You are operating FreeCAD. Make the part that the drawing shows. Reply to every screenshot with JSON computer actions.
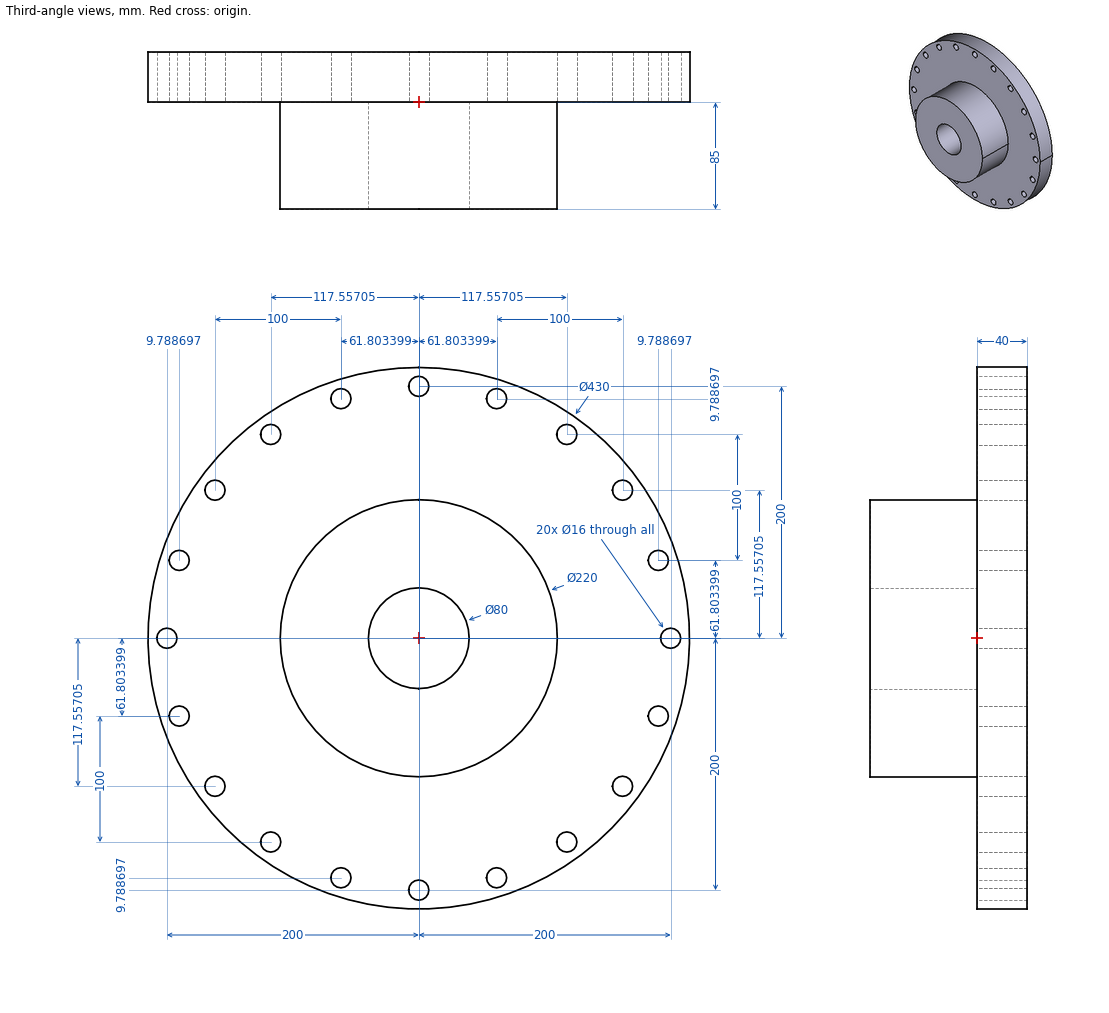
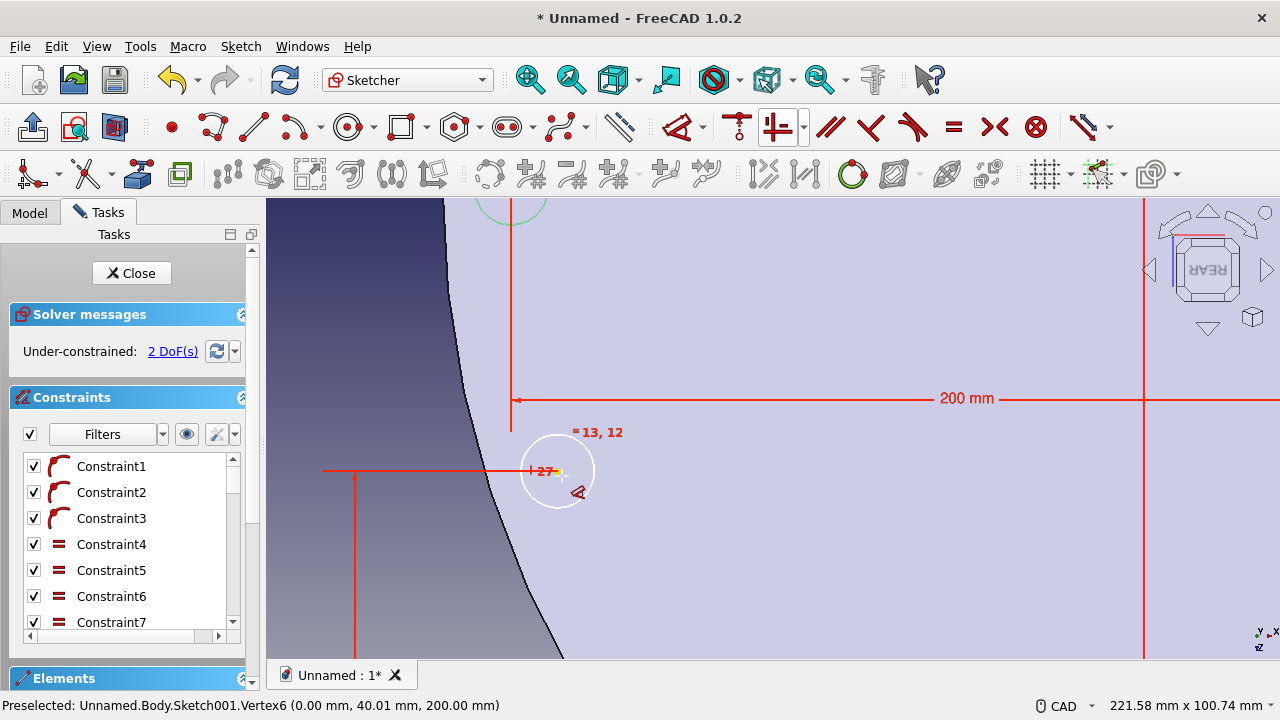
{"action": "left_click", "coordinate": [558, 471]}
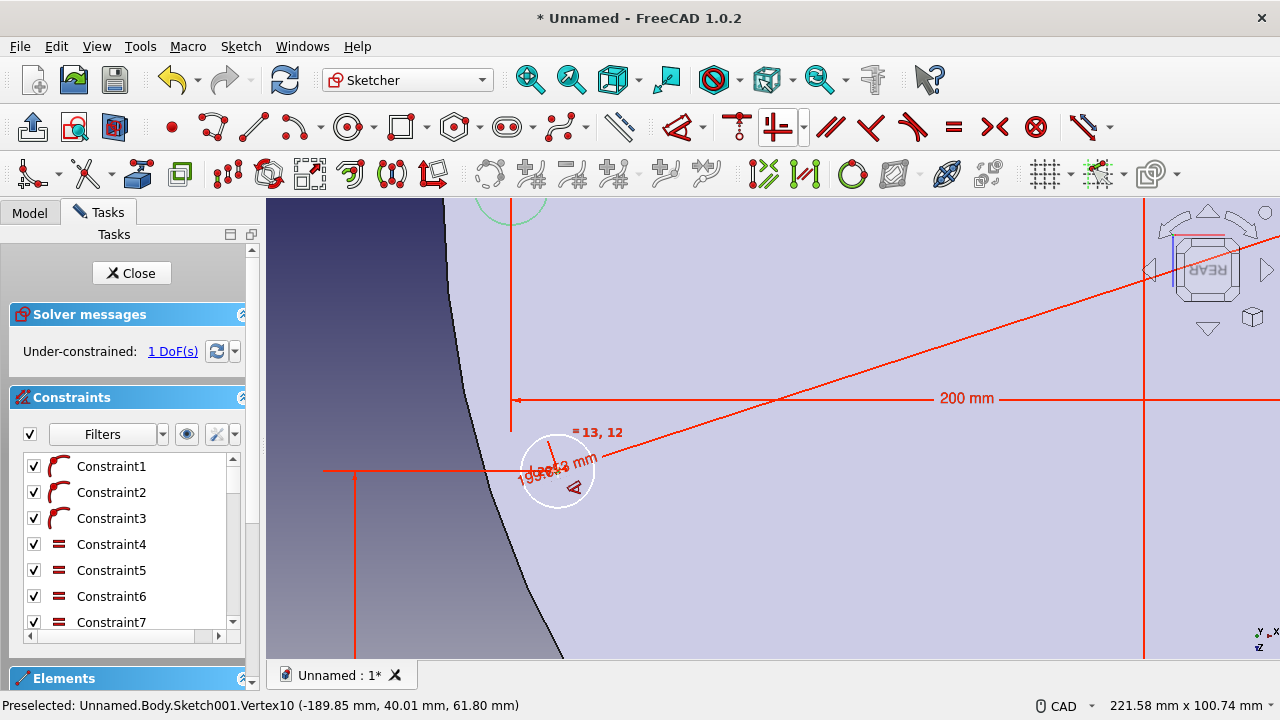
{"action": "scroll", "coordinate": [562, 476], "scroll_direction": "down", "scroll_amount": 9}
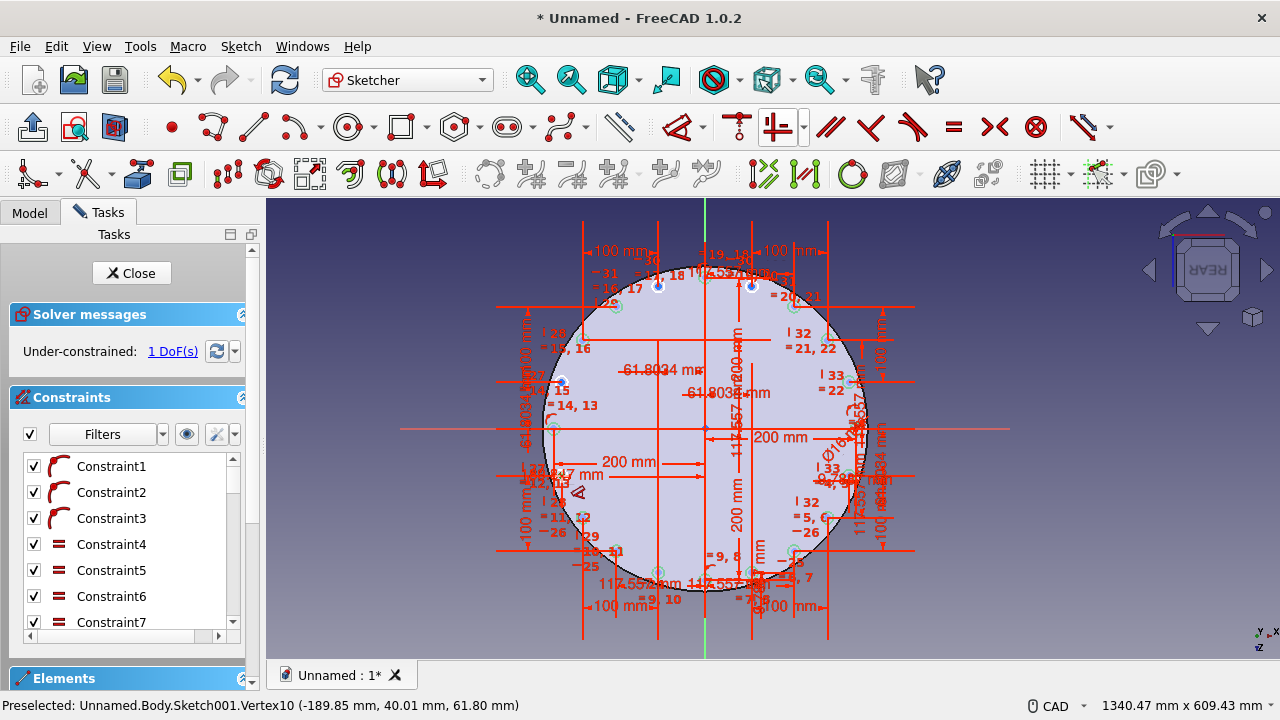
{"action": "scroll", "coordinate": [554, 429], "scroll_direction": "up", "scroll_amount": 9}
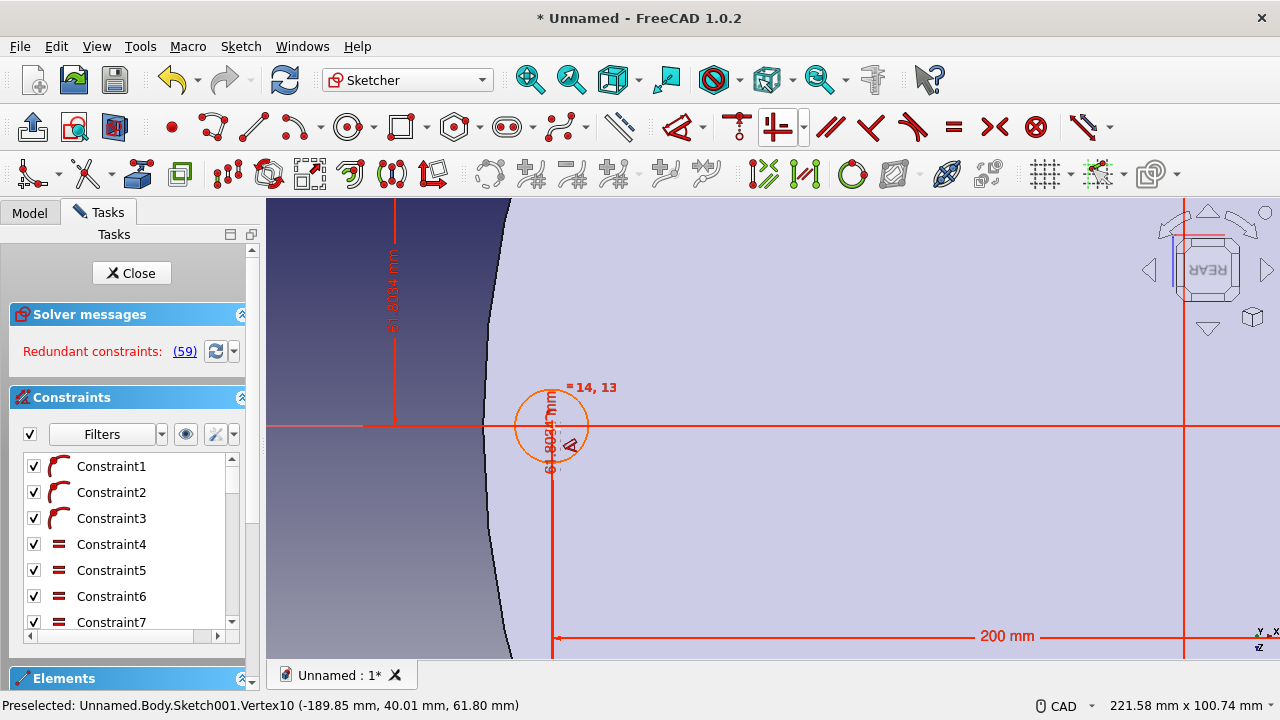
{"action": "left_click", "coordinate": [552, 426]}
{"action": "left_click", "coordinate": [591, 392]}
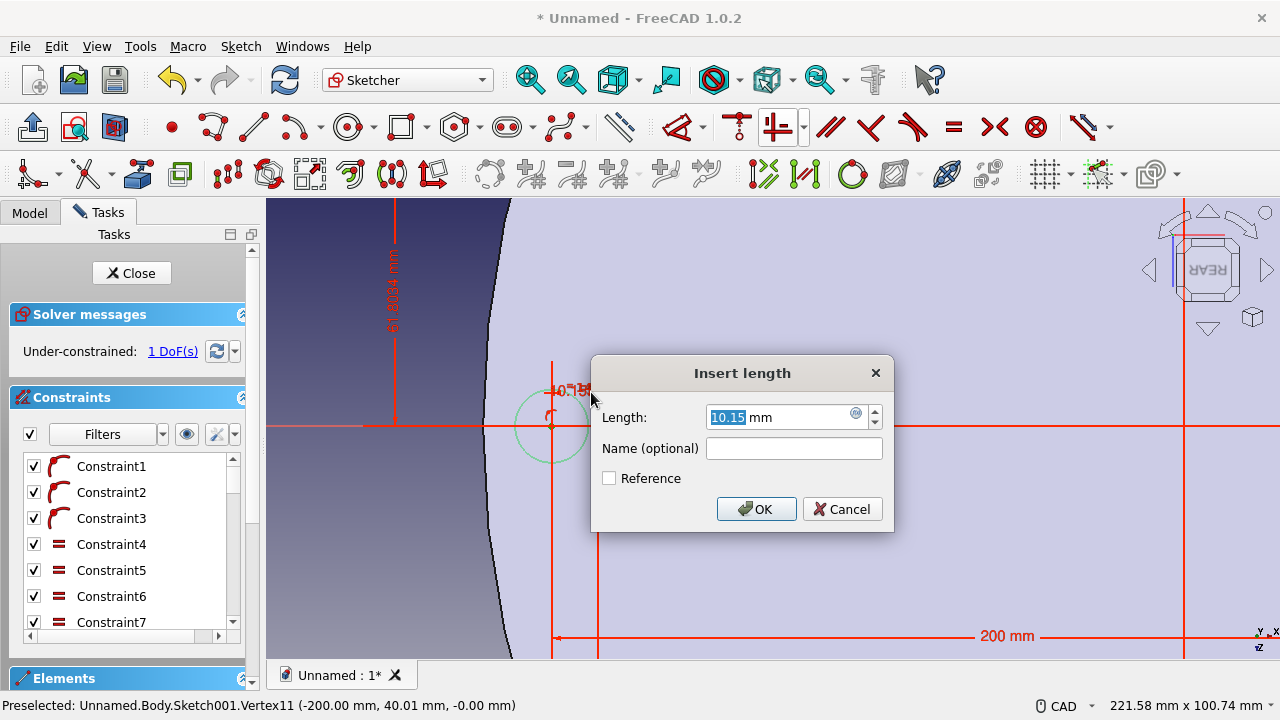
{"action": "type", "text": "9.788697"}
{"action": "key", "text": "Return"}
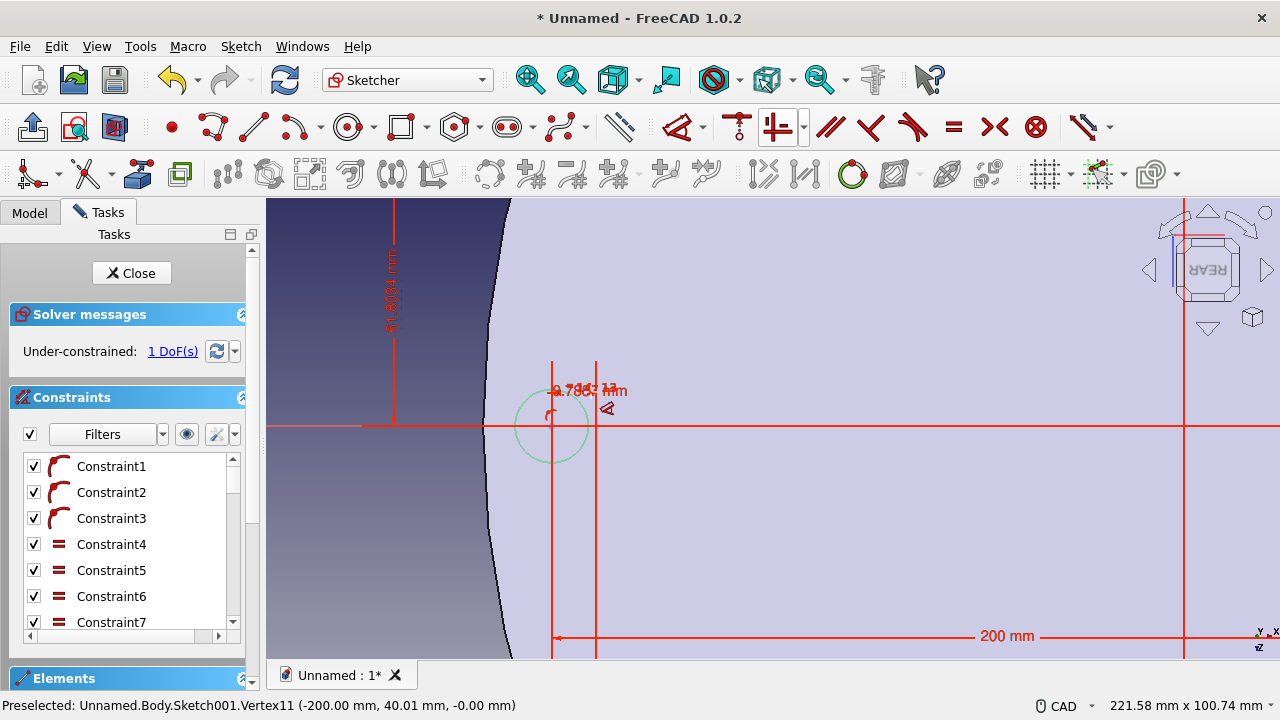
{"action": "scroll", "coordinate": [554, 429], "scroll_direction": "down", "scroll_amount": 9}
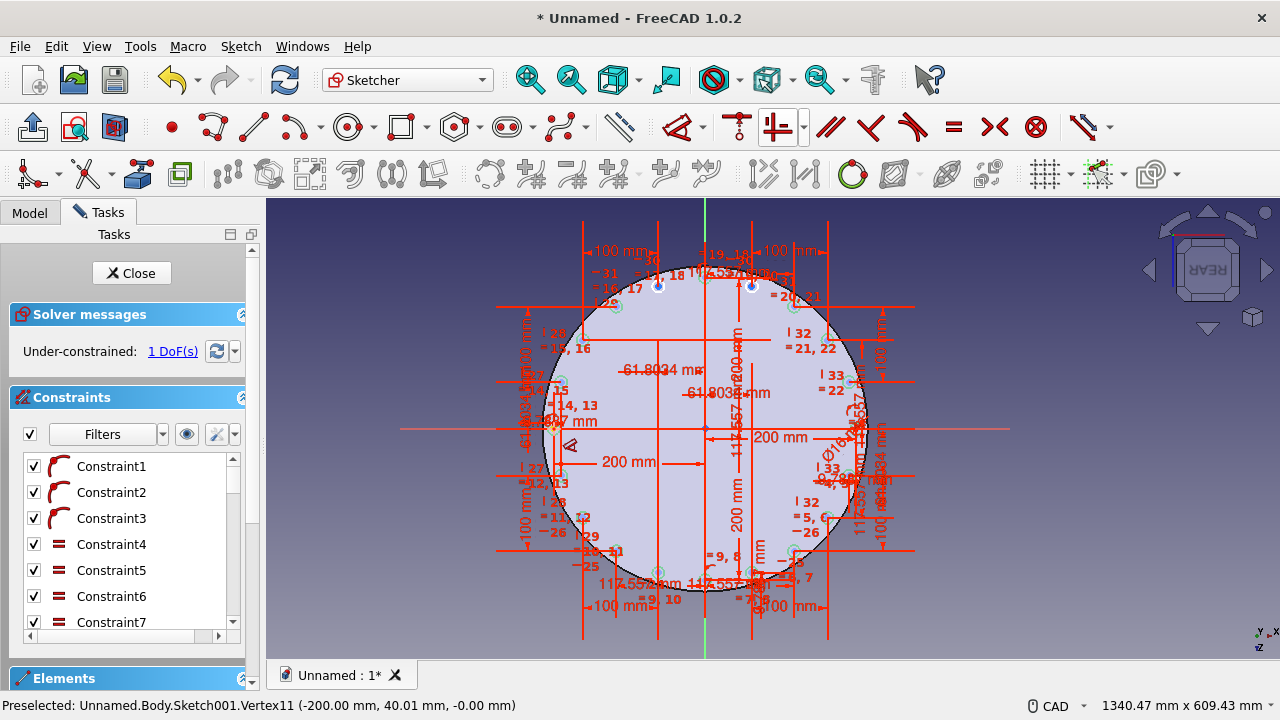
{"action": "scroll", "coordinate": [658, 286], "scroll_direction": "up", "scroll_amount": 9}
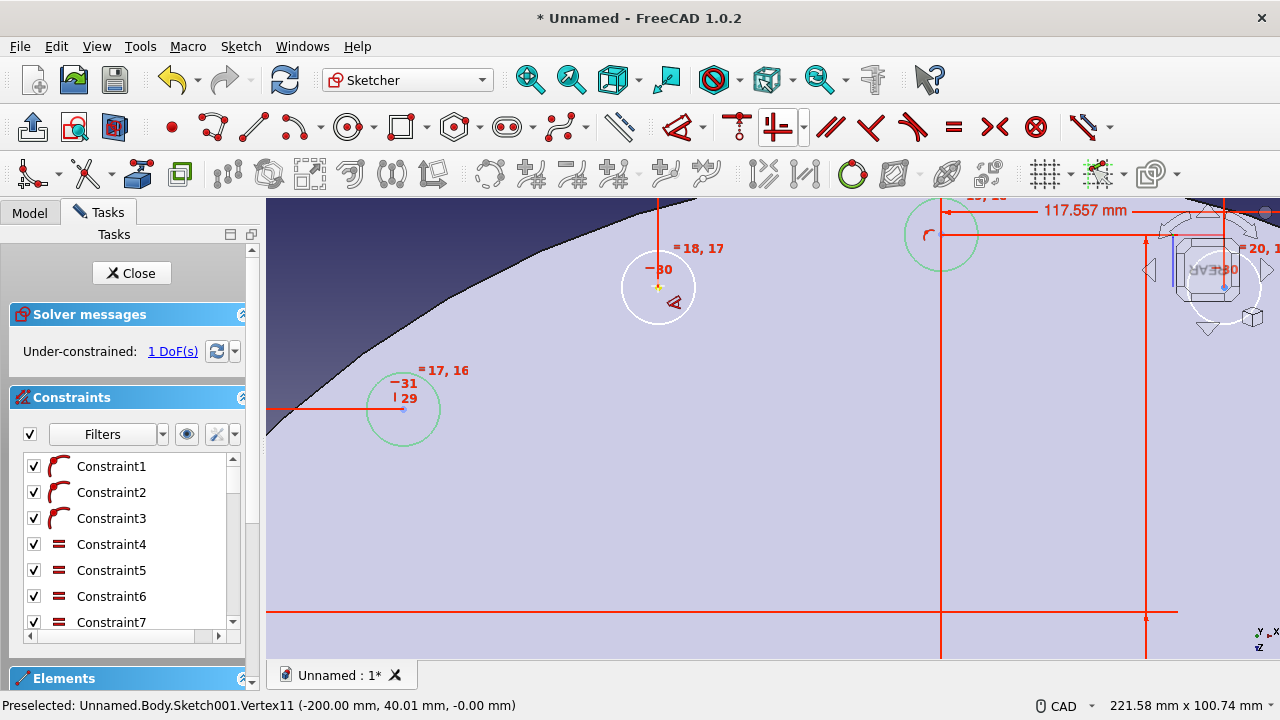
{"action": "left_click", "coordinate": [658, 287]}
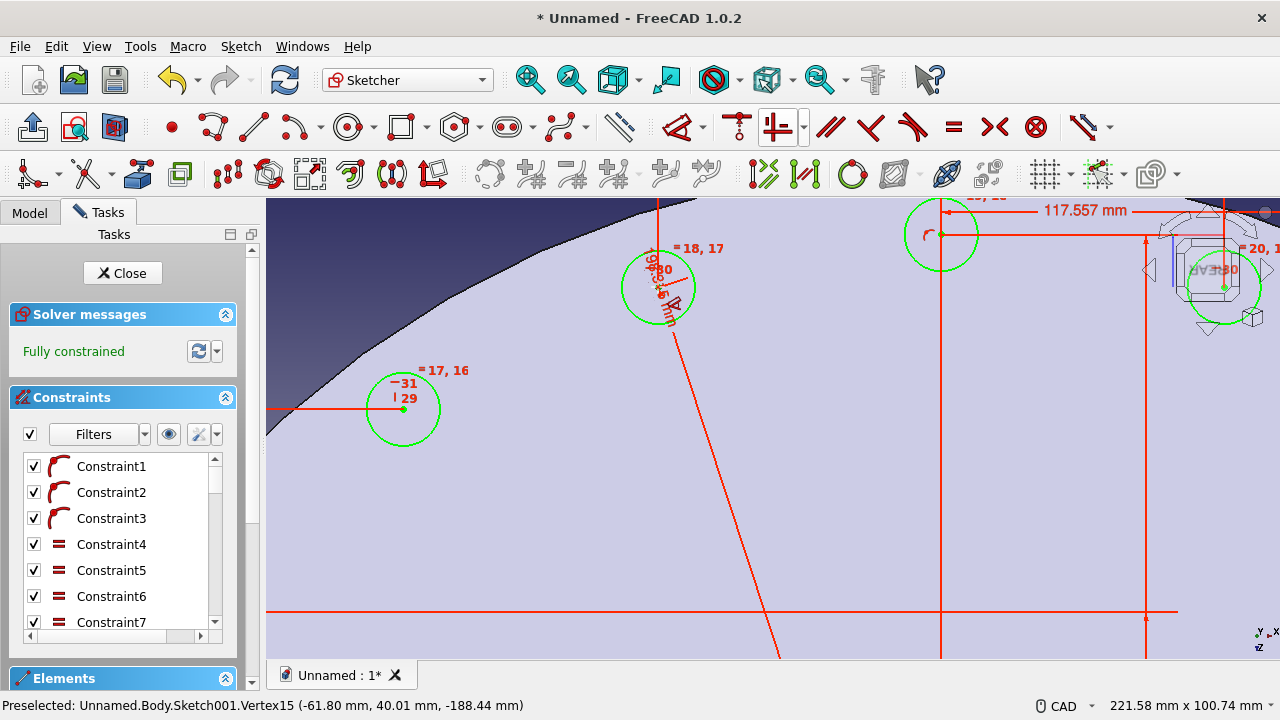
{"action": "left_click", "coordinate": [941, 235]}
{"action": "left_click", "coordinate": [624, 249]}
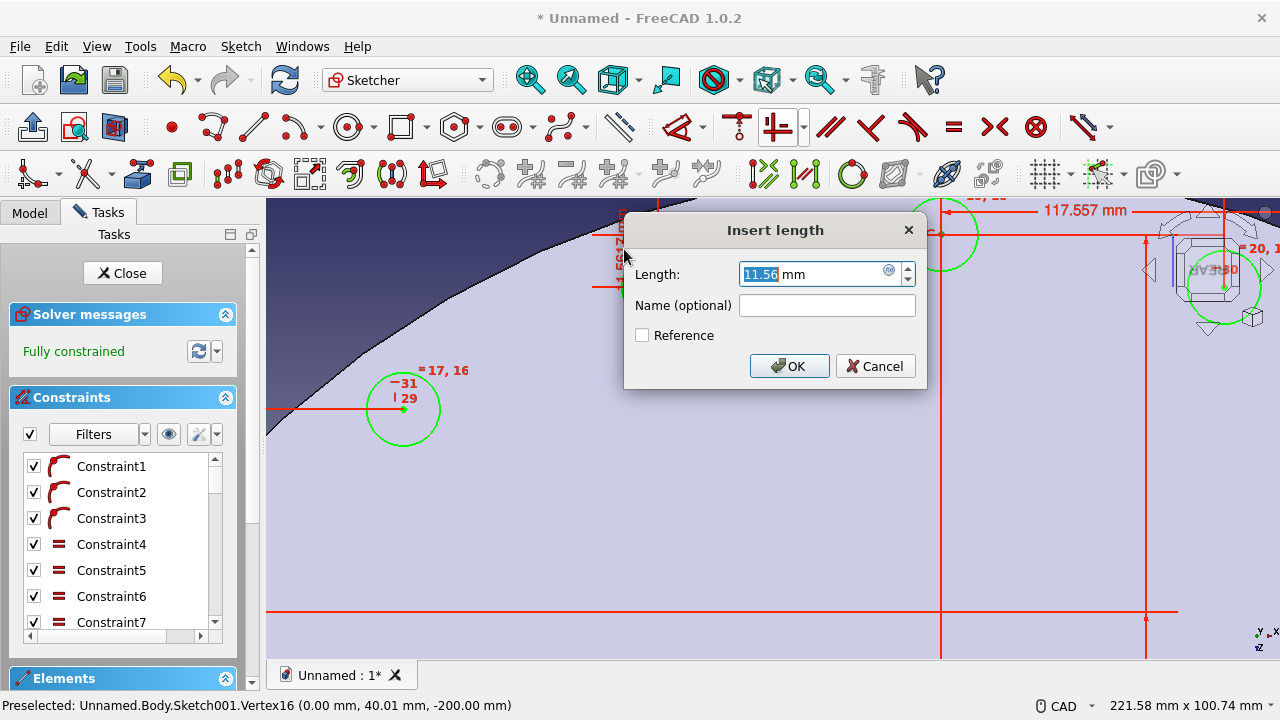
{"action": "type", "text": "9.788697"}
{"action": "key", "text": "Return"}
{"action": "key", "text": "Escape"}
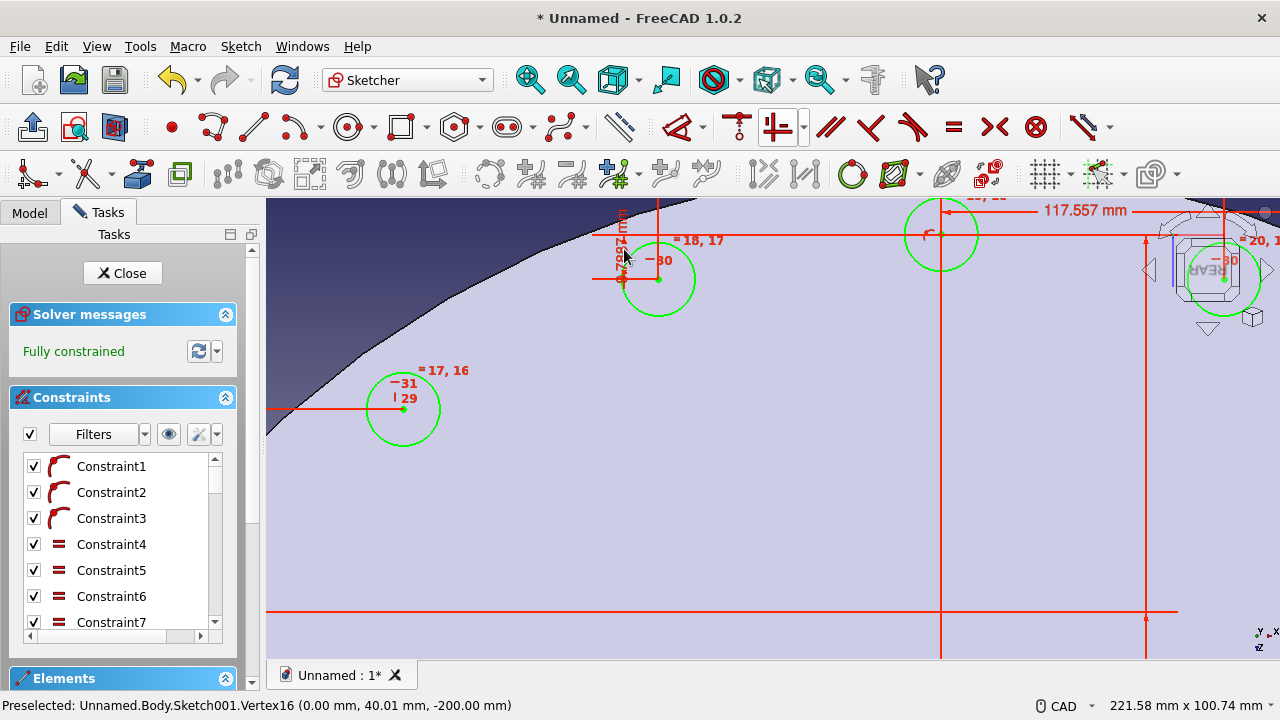
{"action": "left_click", "coordinate": [123, 273]}